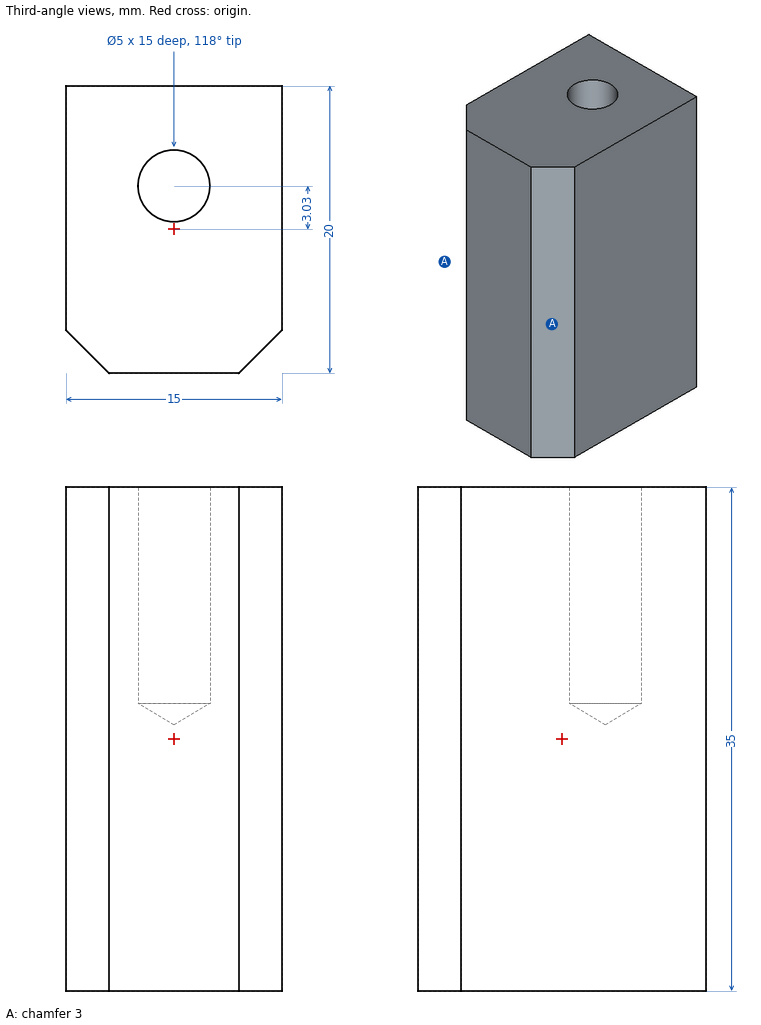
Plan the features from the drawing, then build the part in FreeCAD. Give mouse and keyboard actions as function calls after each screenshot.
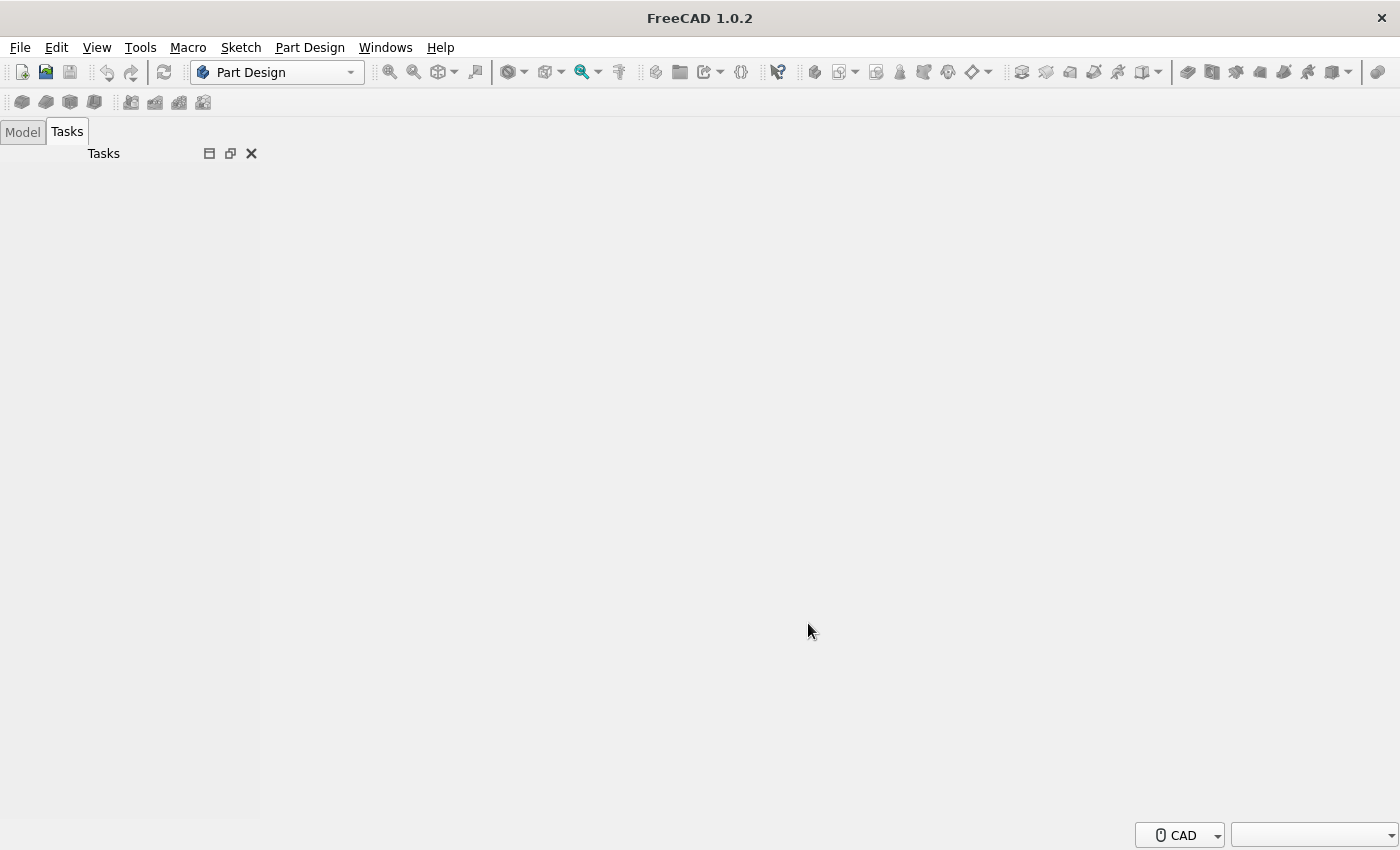
click(22, 72)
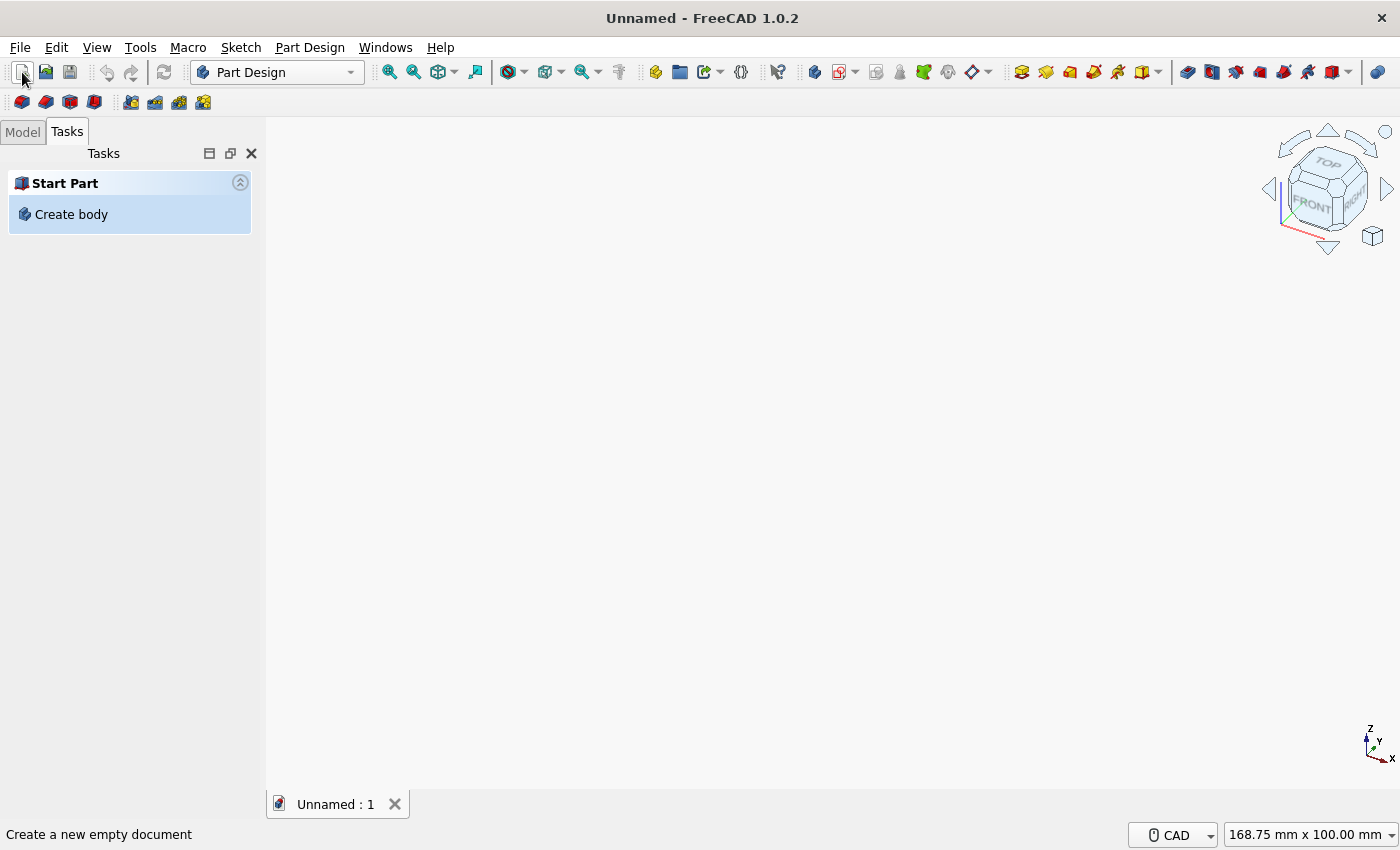
click(840, 72)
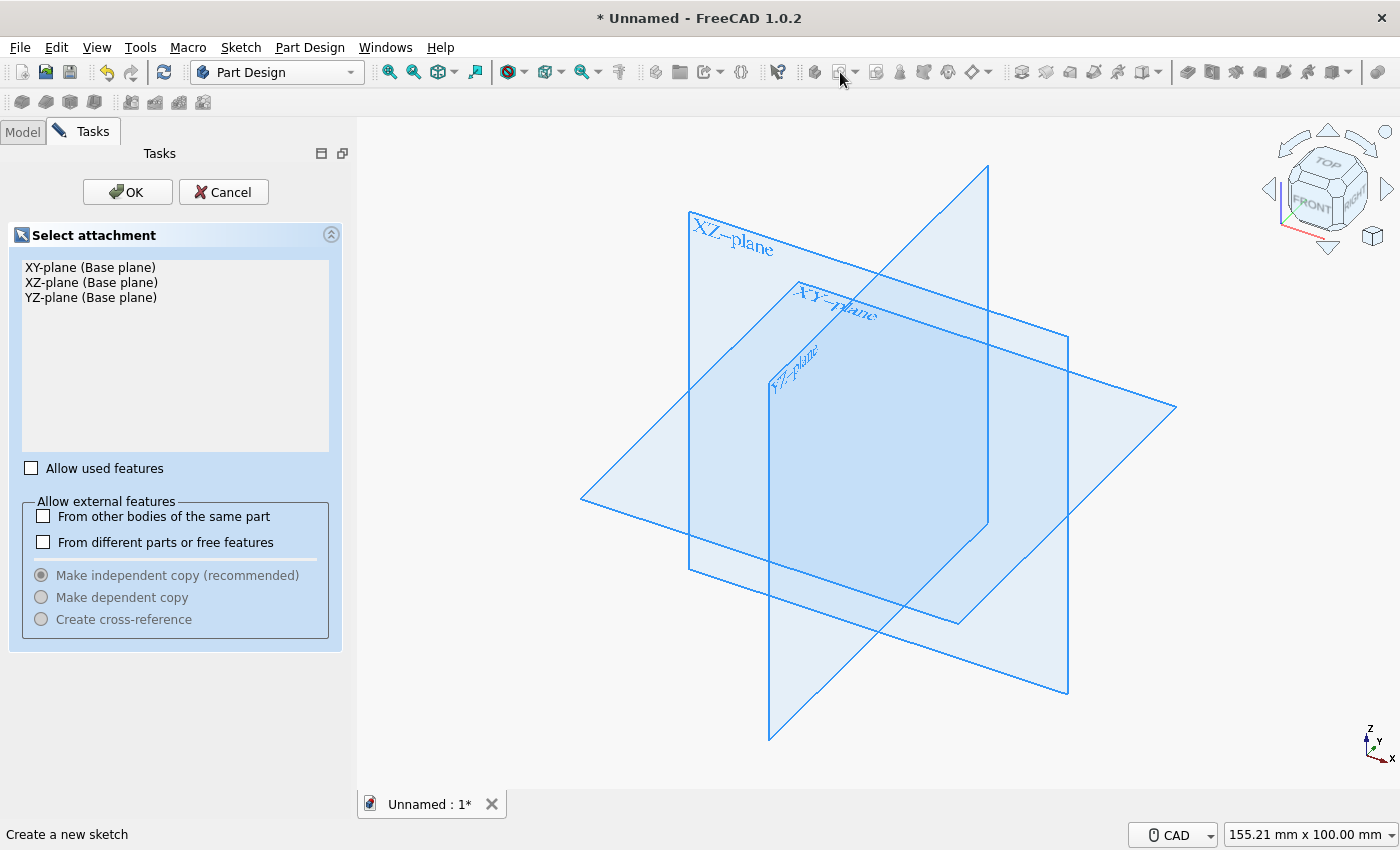
click(82, 268)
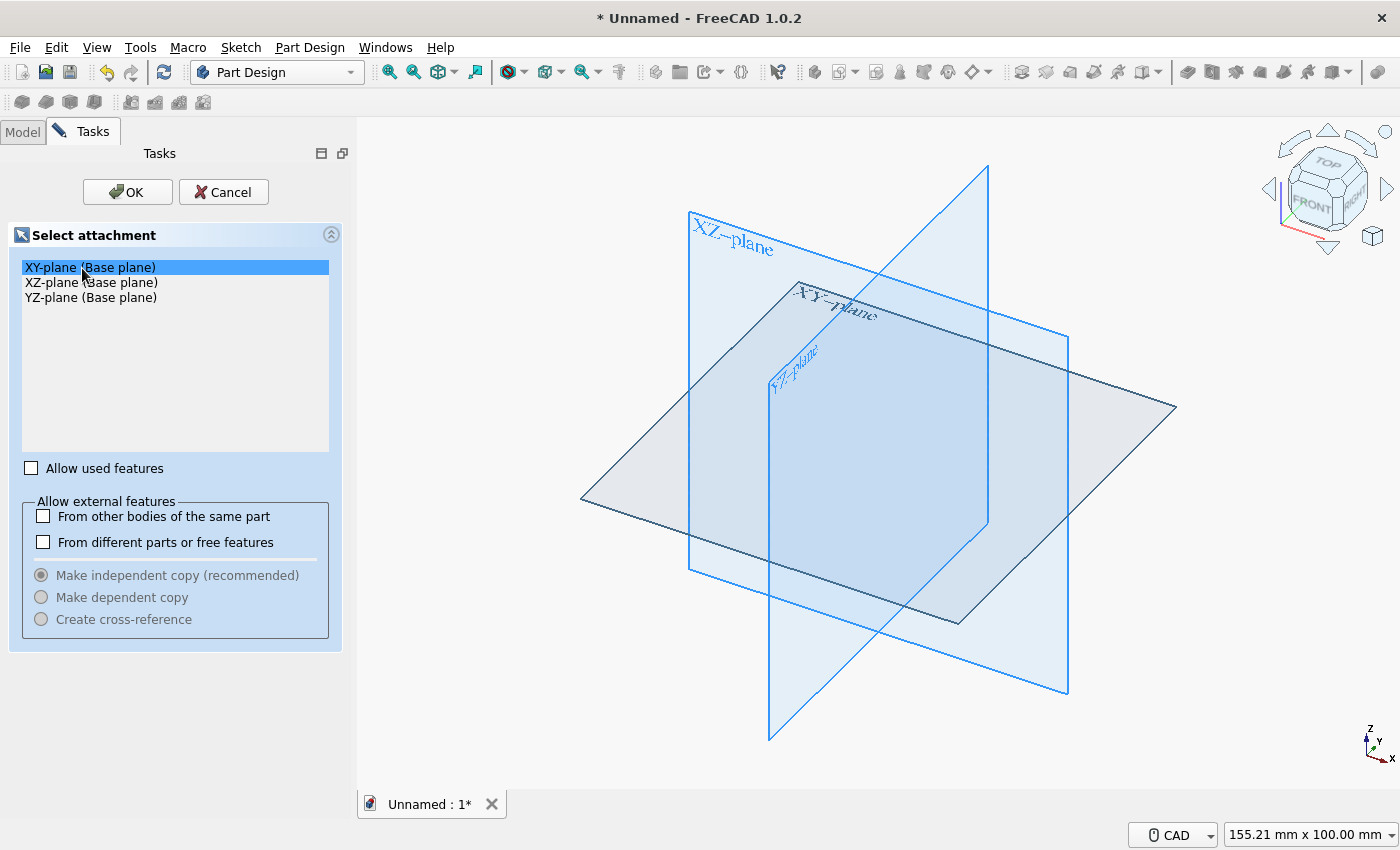
click(128, 192)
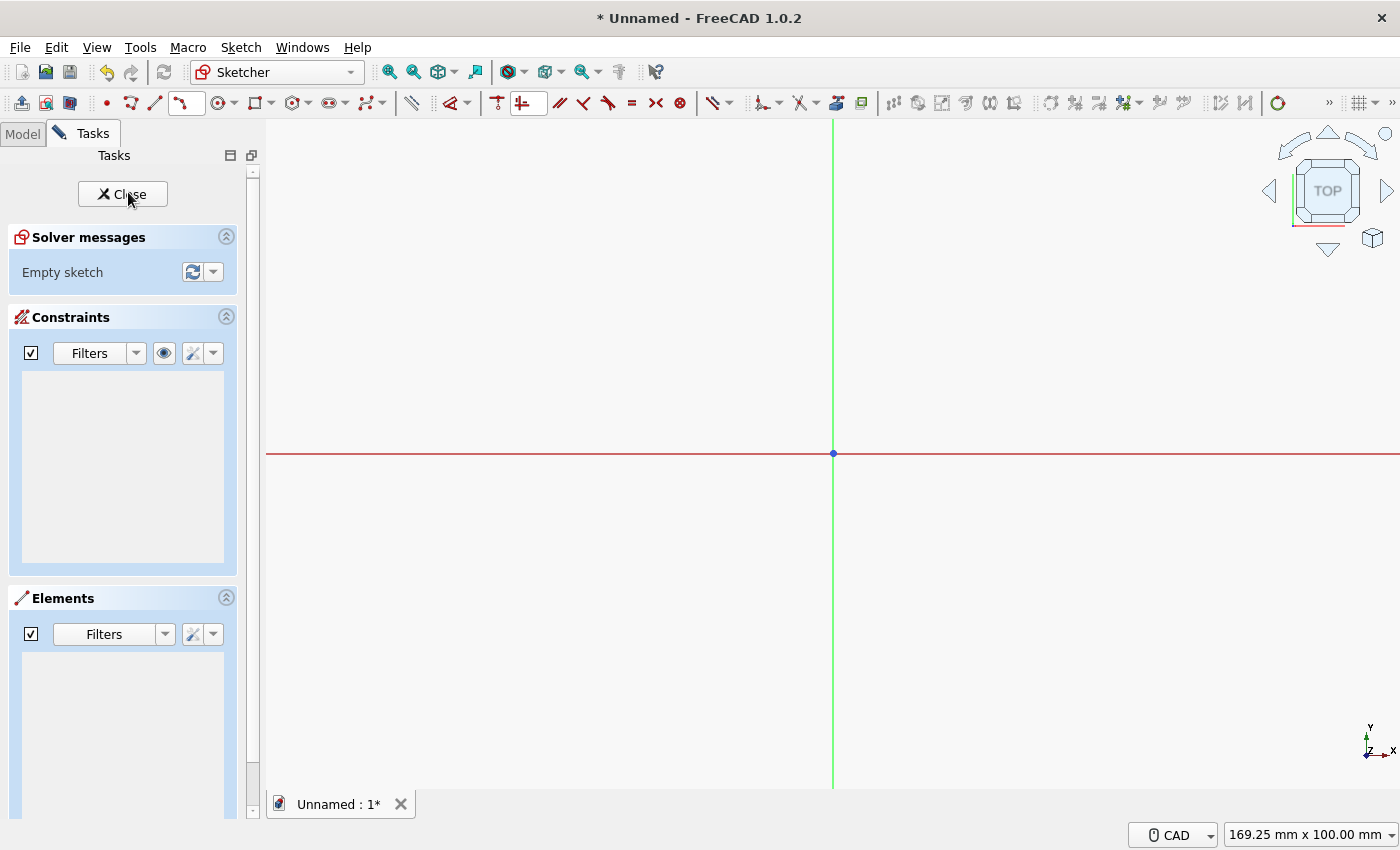
scroll(863, 454, up, 6)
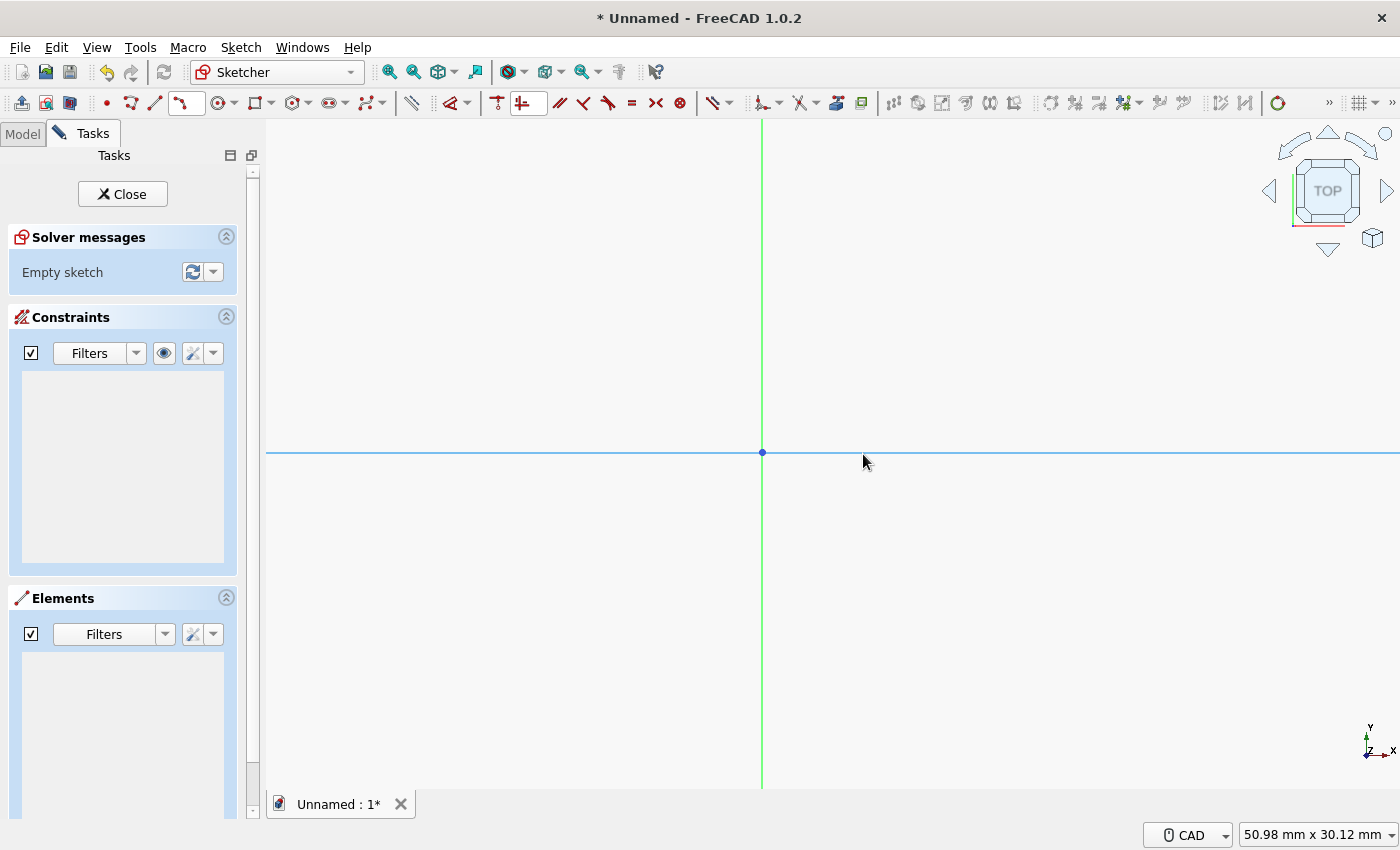
click(274, 104)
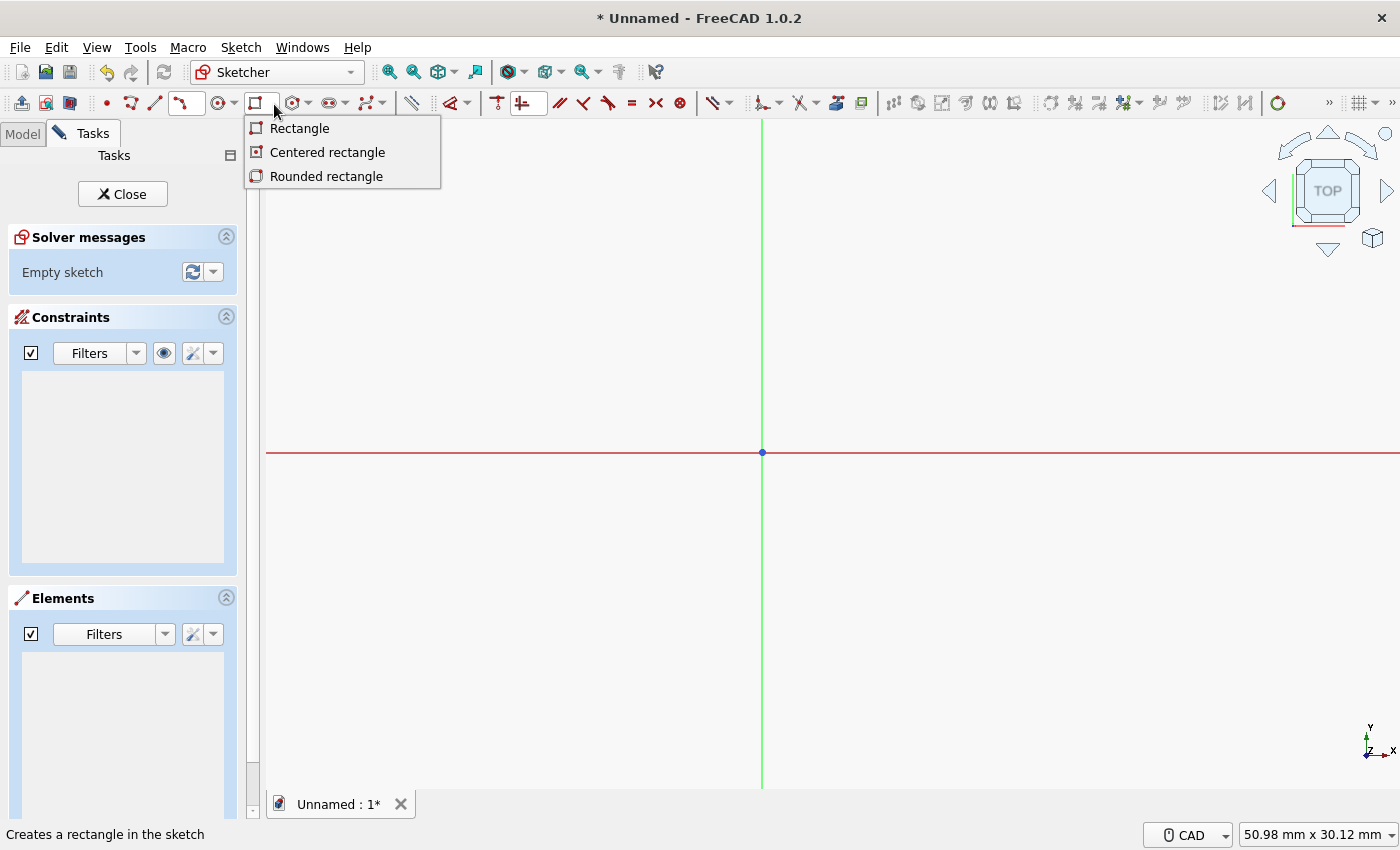
click(342, 152)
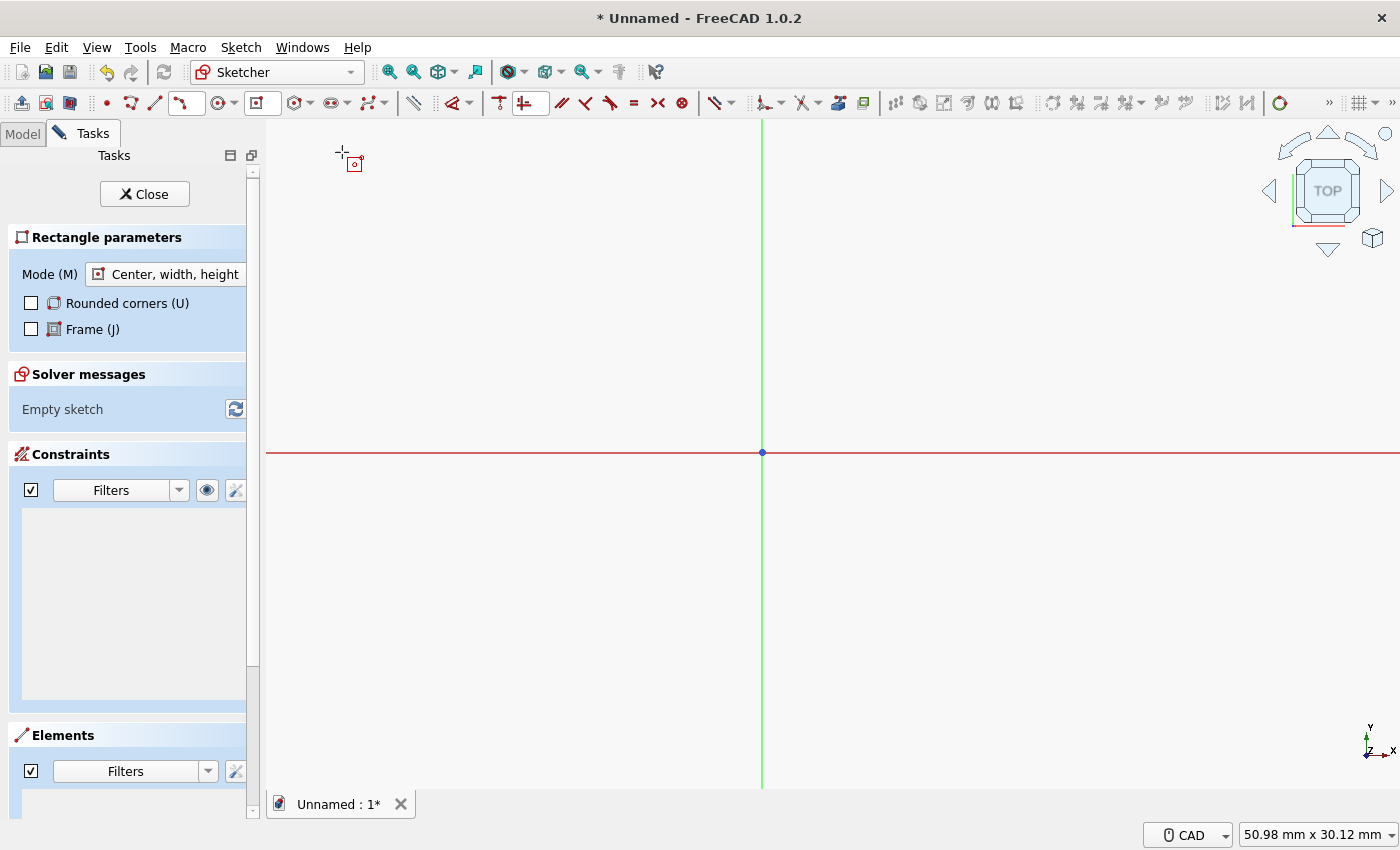
click(762, 453)
move(929, 230)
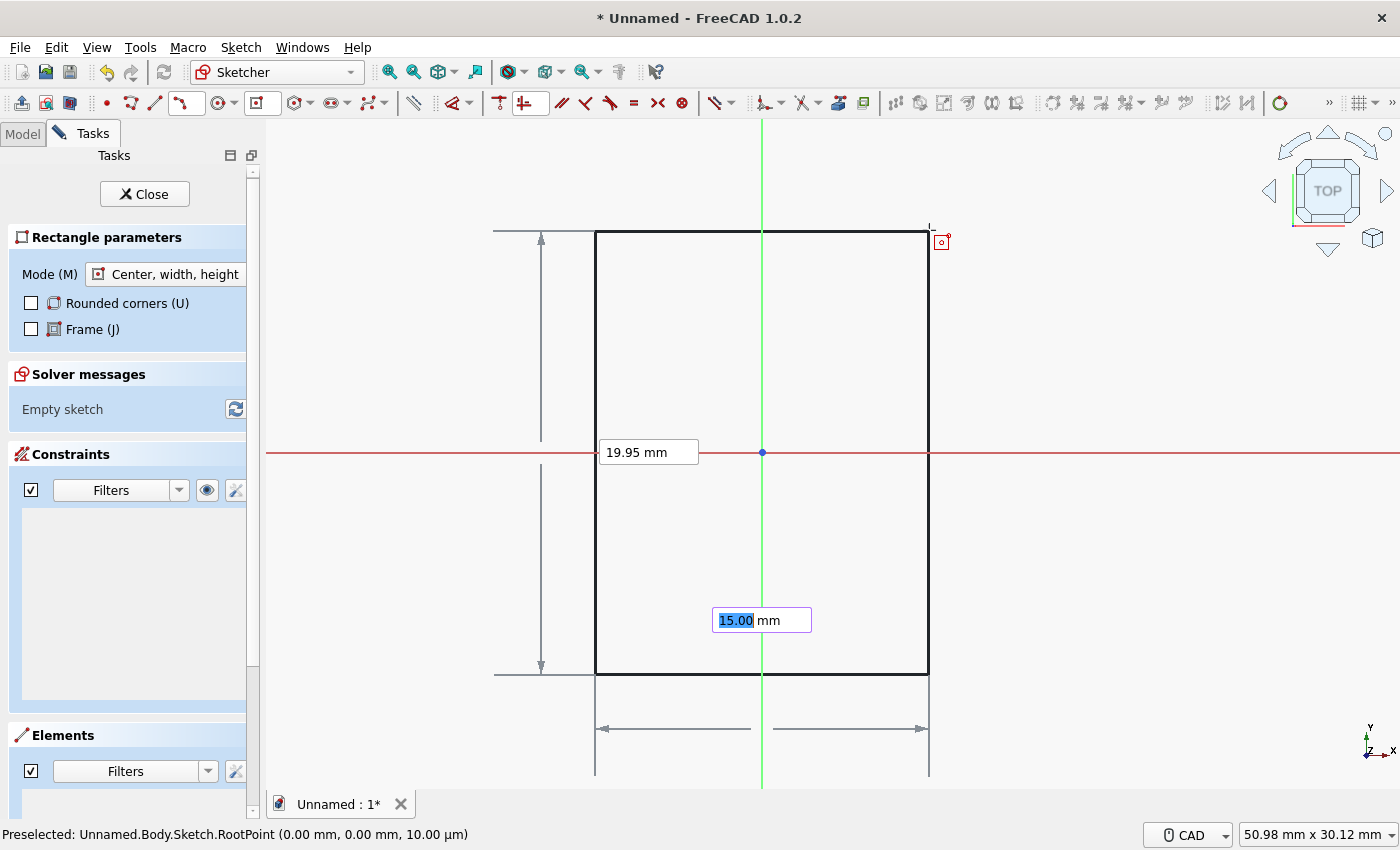
text(15)
key(Tab)
text(20)
key(Return)
key(Escape)